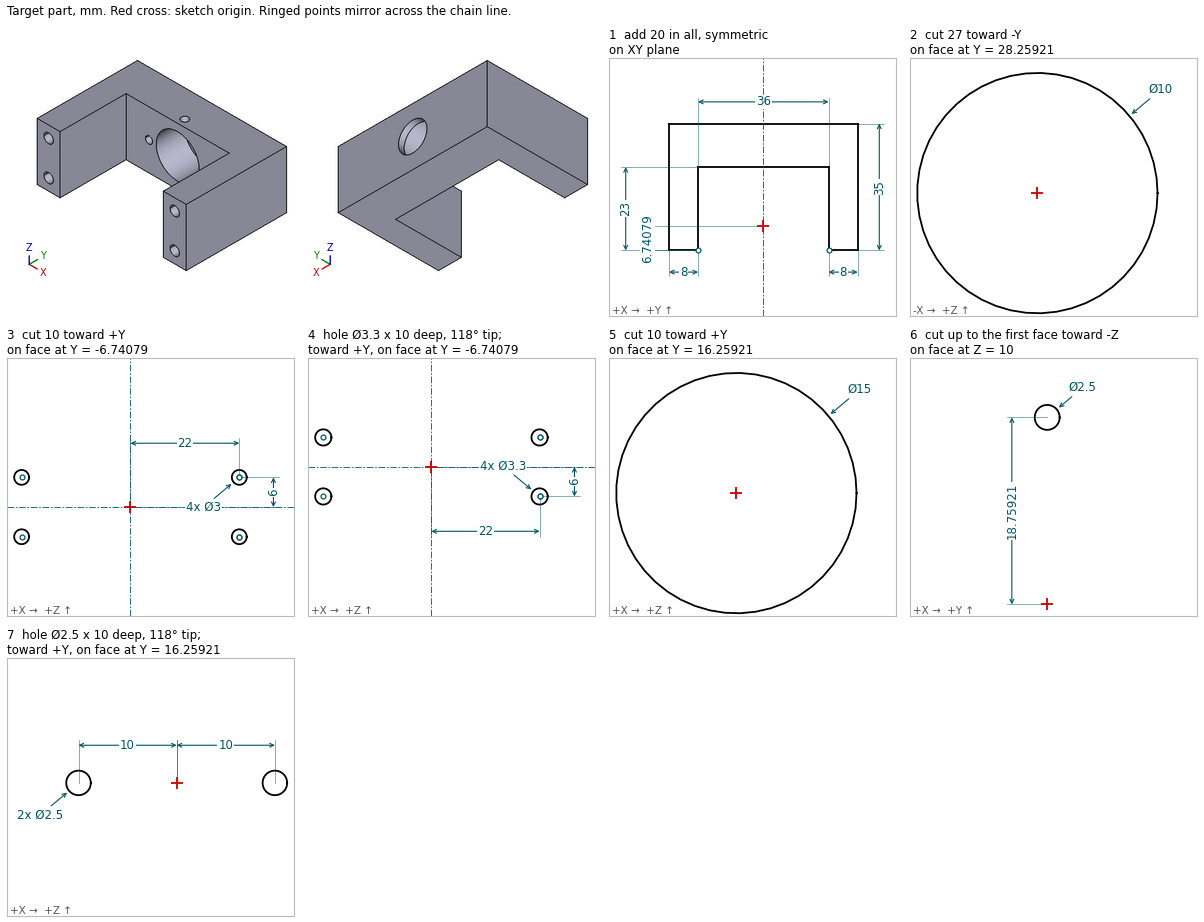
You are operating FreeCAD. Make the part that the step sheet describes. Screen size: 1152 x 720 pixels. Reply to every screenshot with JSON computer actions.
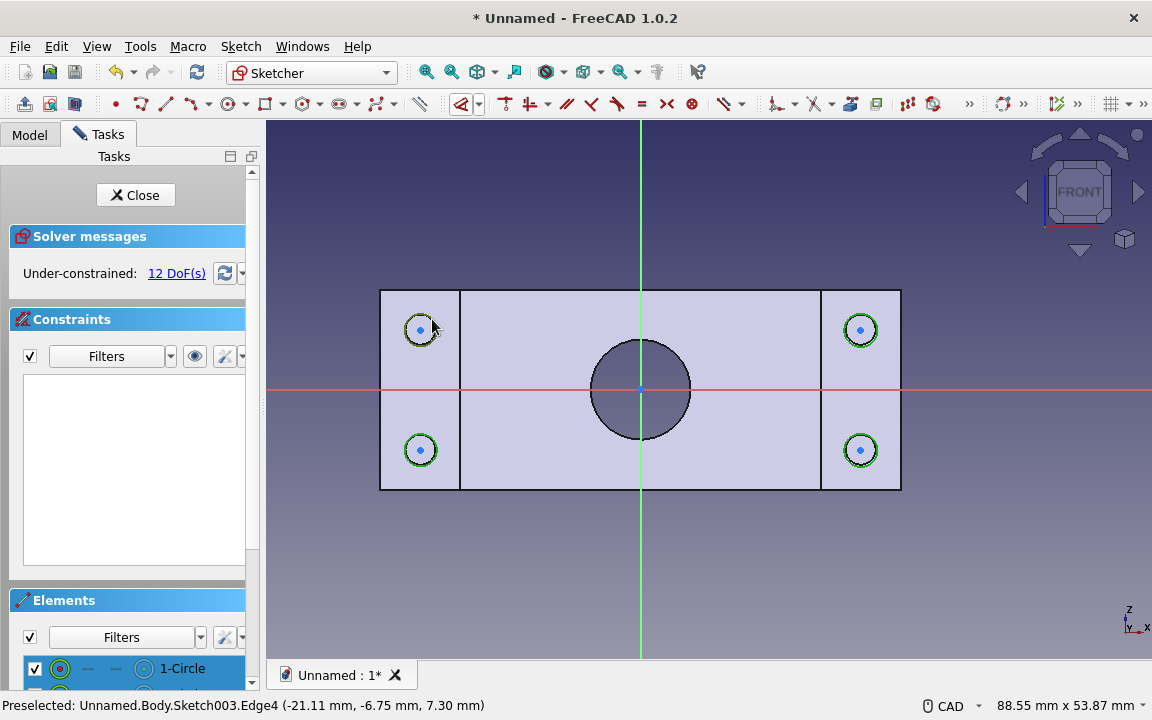
{"action": "key", "text": "e"}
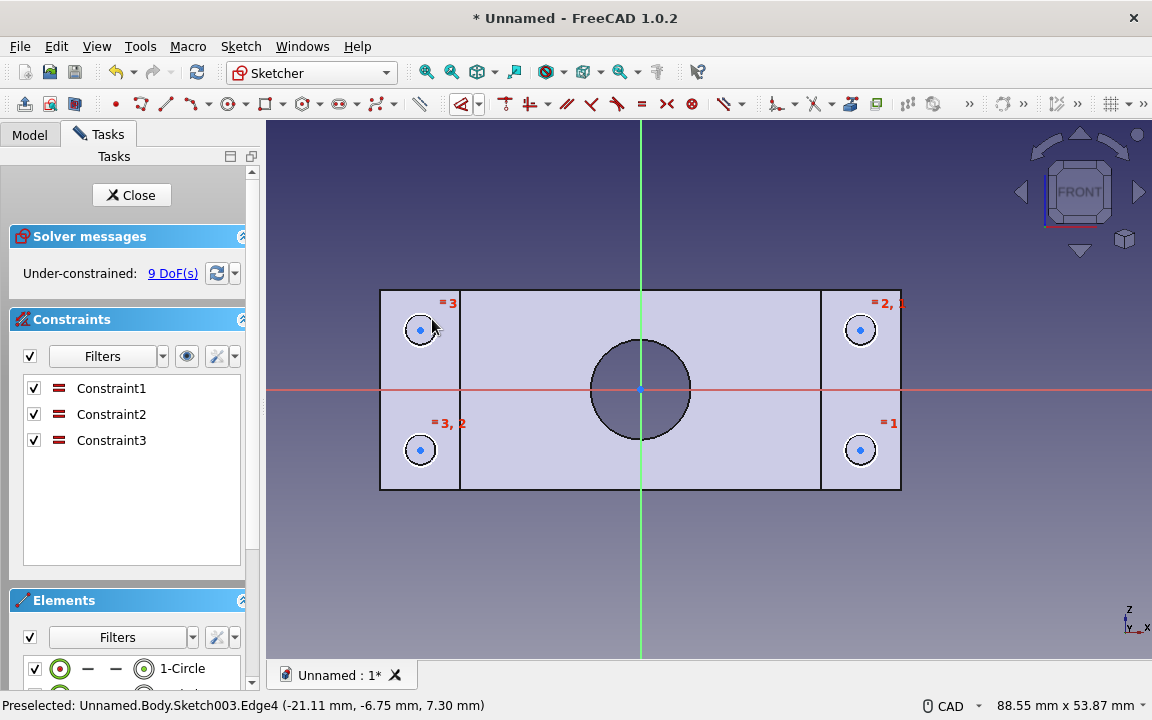
{"action": "left_click", "coordinate": [861, 450]}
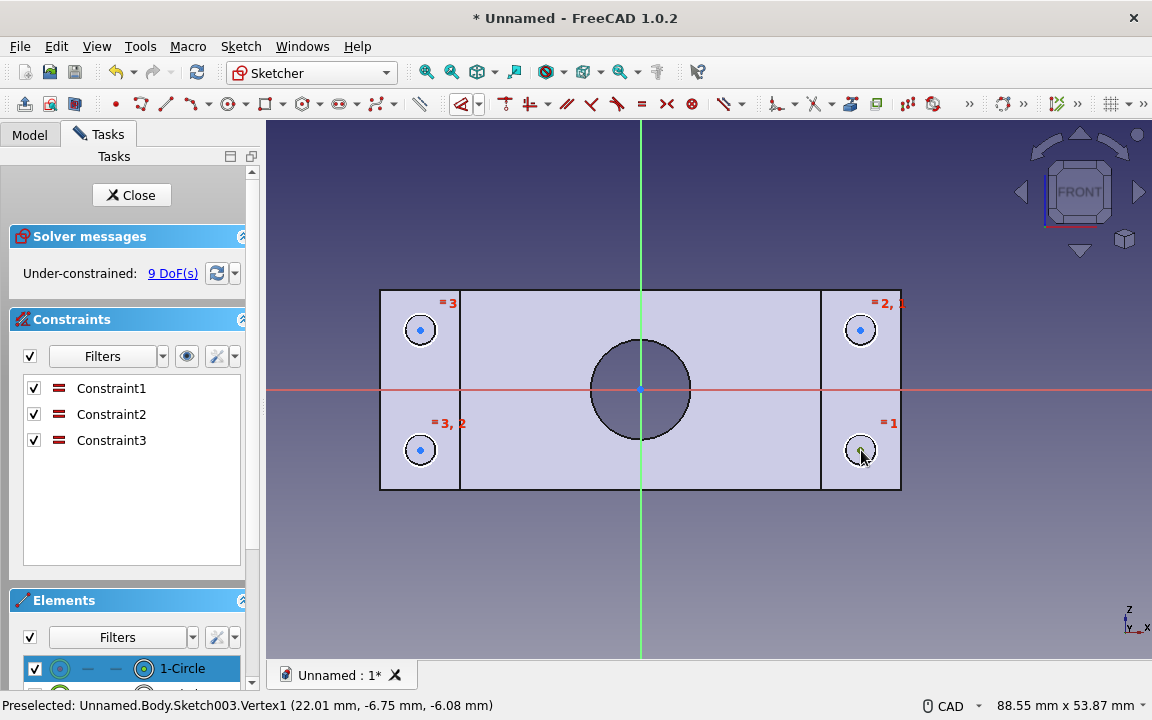
{"action": "left_click", "coordinate": [861, 330]}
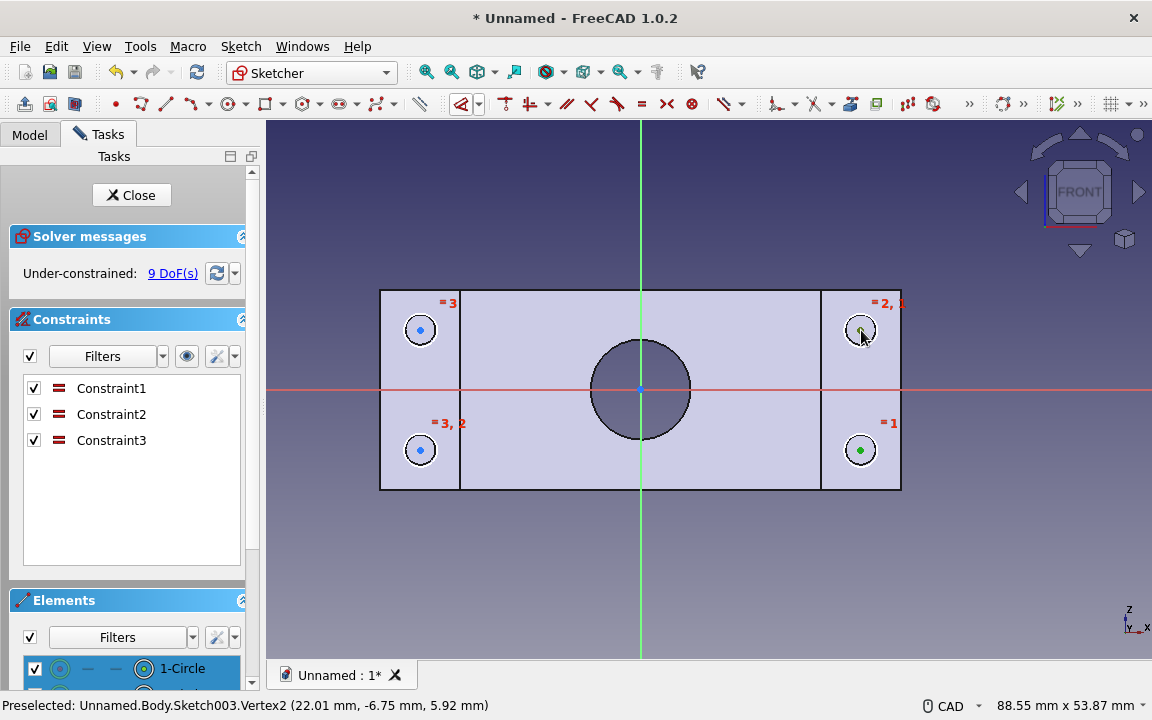
{"action": "left_click", "coordinate": [344, 390]}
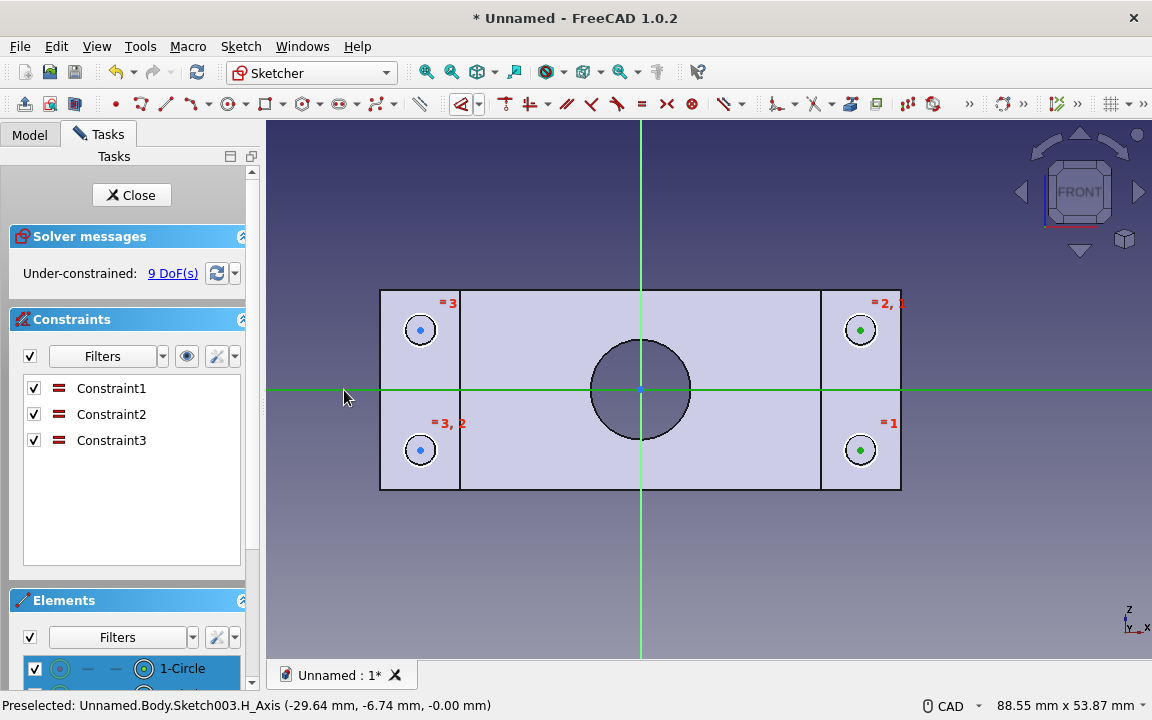
{"action": "key", "text": "s"}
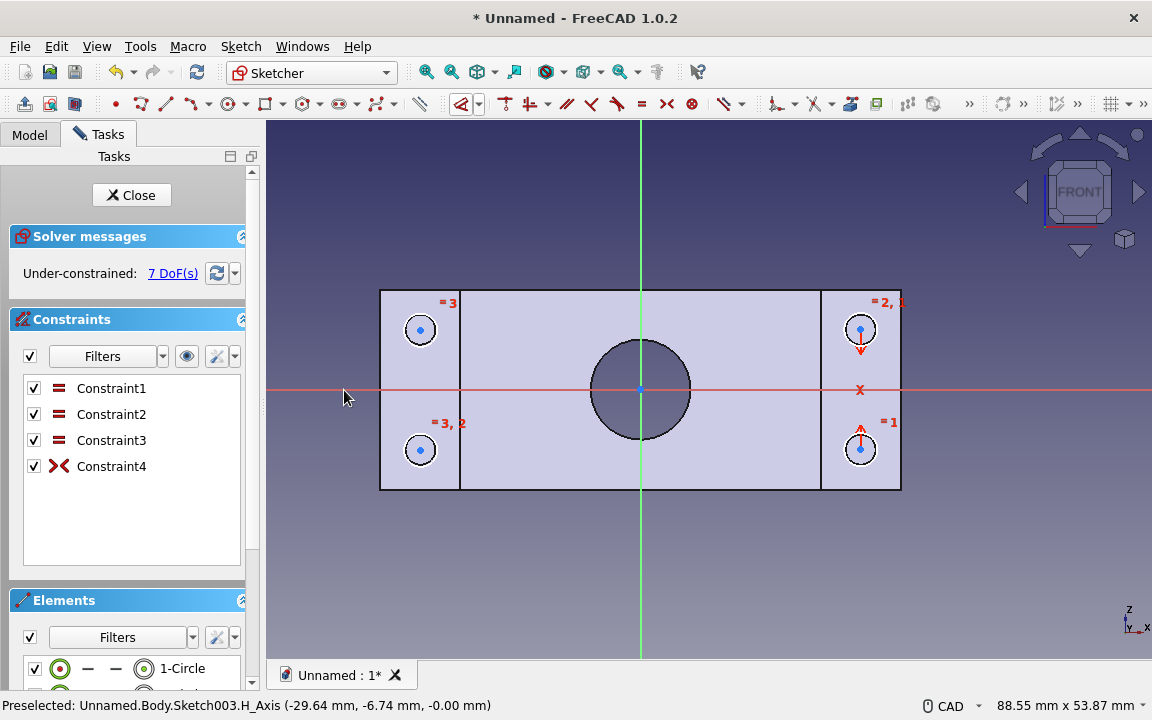
{"action": "left_click", "coordinate": [861, 450]}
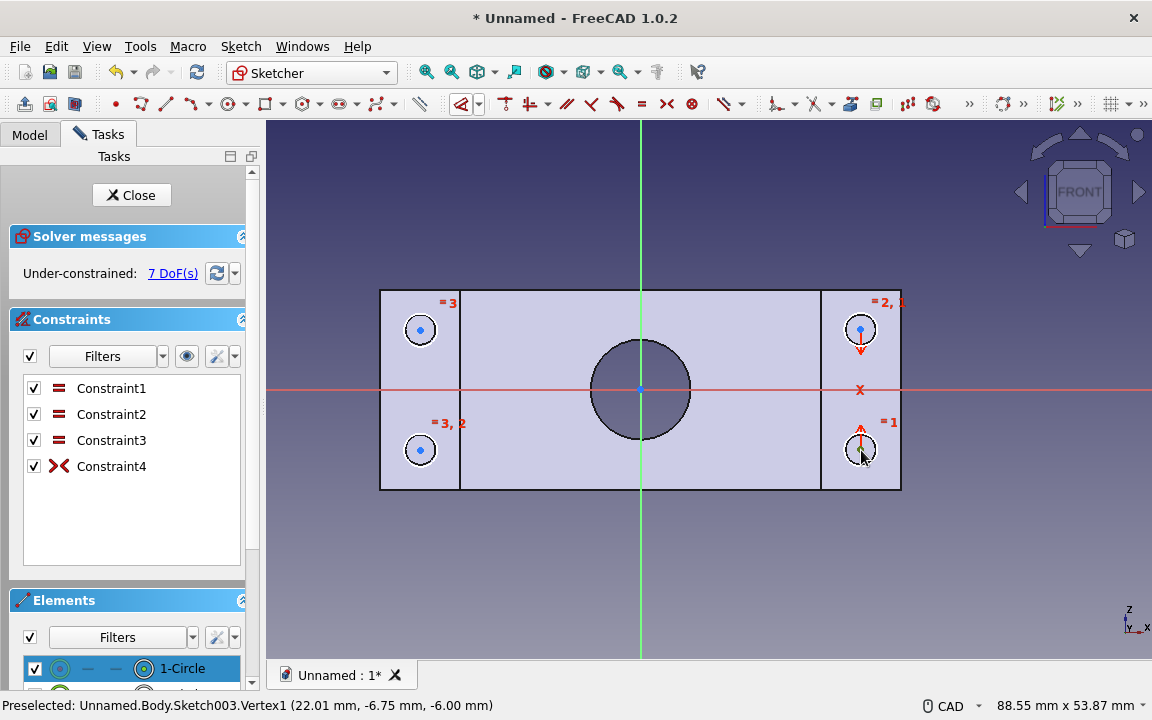
{"action": "left_click", "coordinate": [421, 450]}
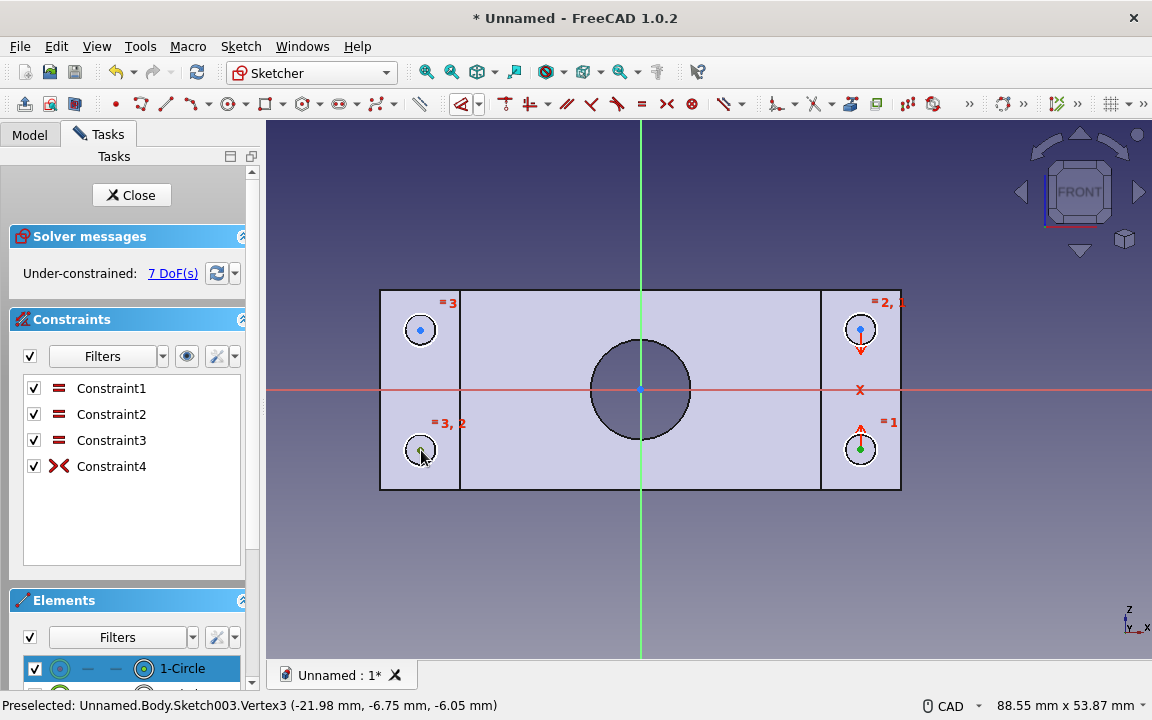
{"action": "left_click", "coordinate": [641, 596]}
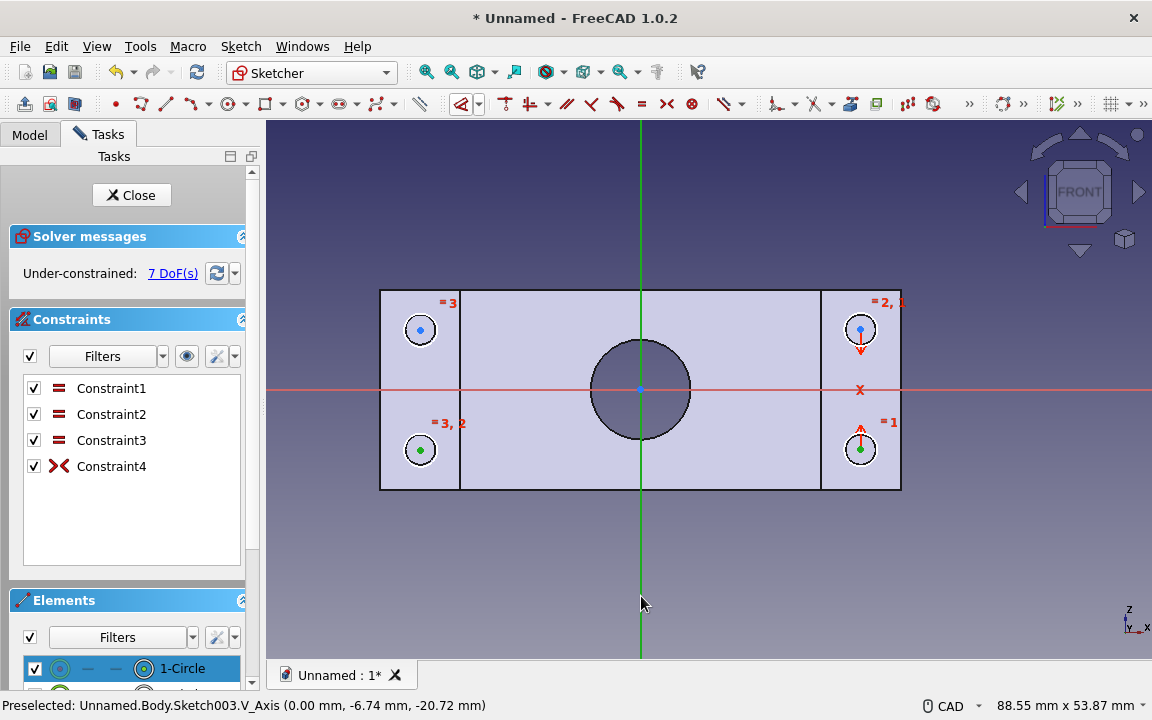
{"action": "key", "text": "s"}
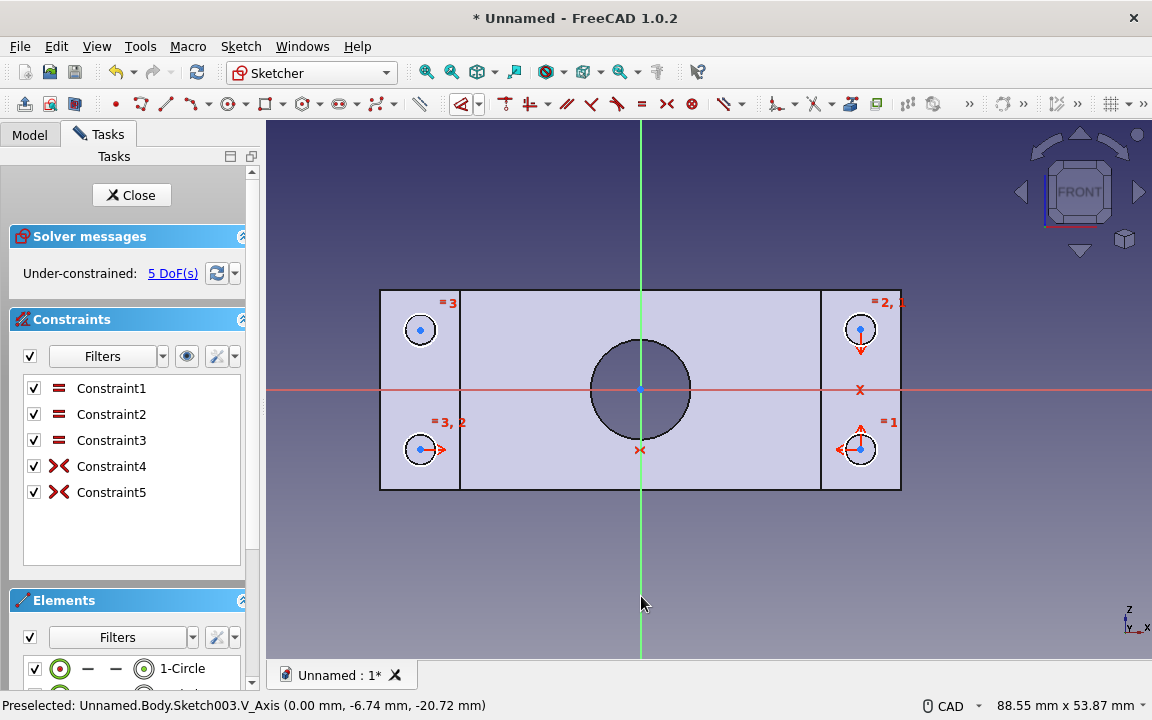
{"action": "left_click", "coordinate": [861, 330]}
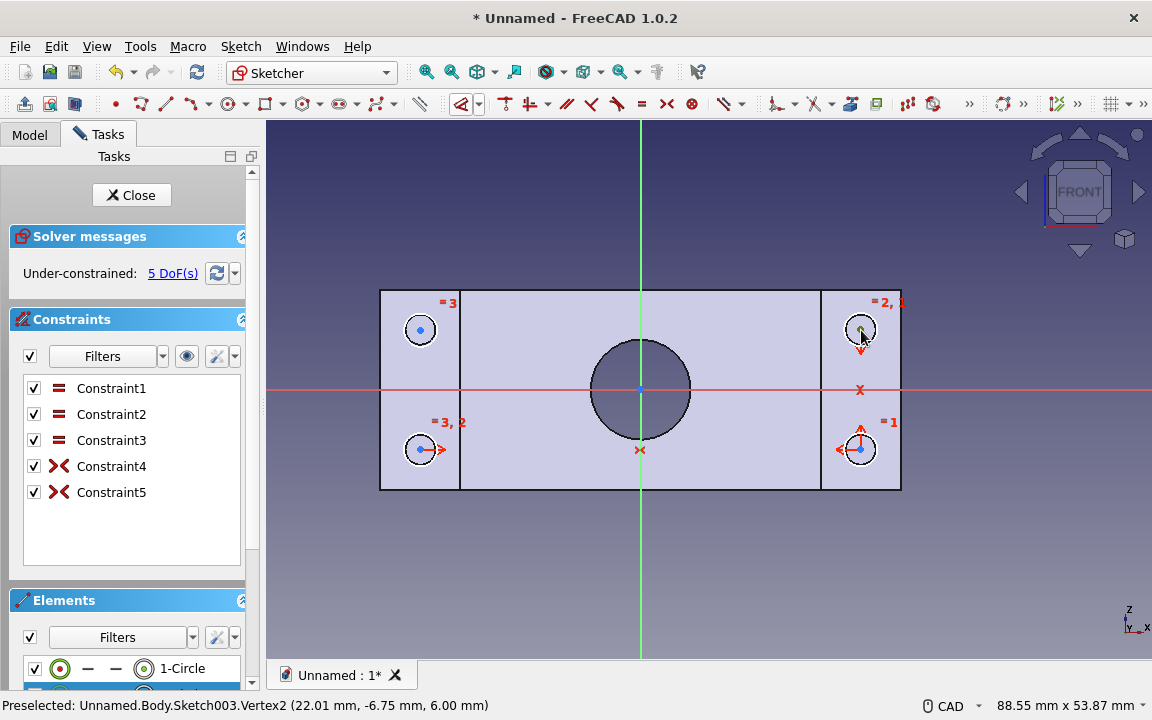
{"action": "left_click", "coordinate": [421, 330]}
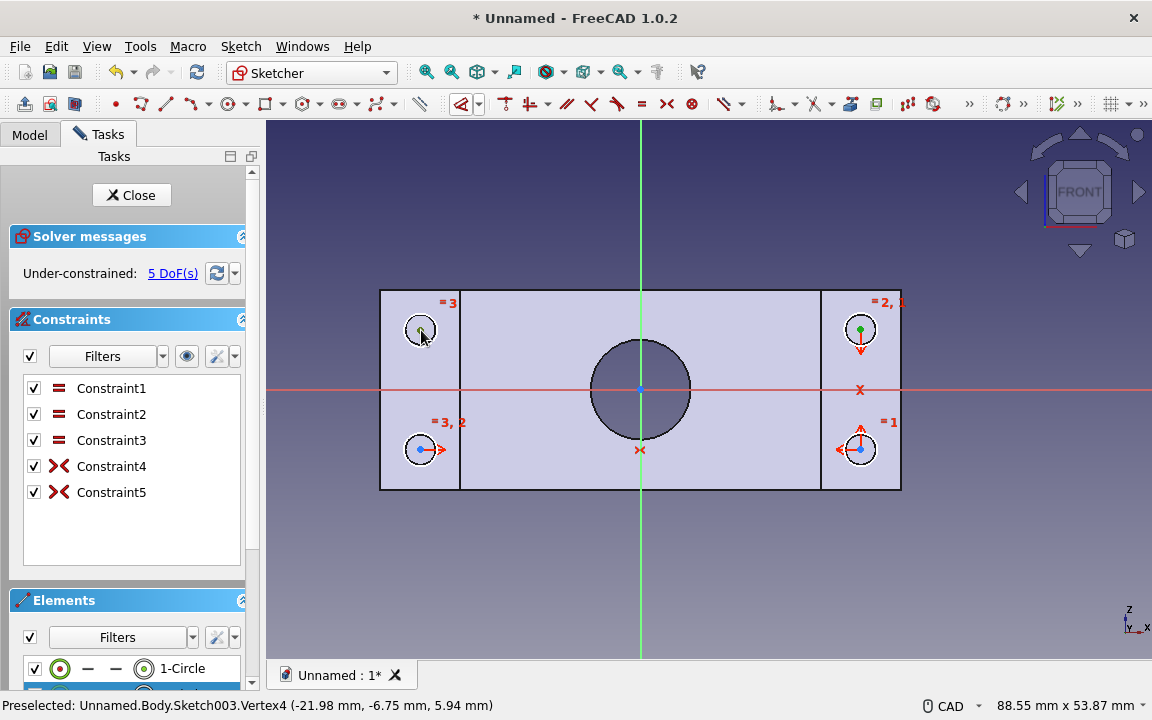
{"action": "left_click", "coordinate": [641, 596]}